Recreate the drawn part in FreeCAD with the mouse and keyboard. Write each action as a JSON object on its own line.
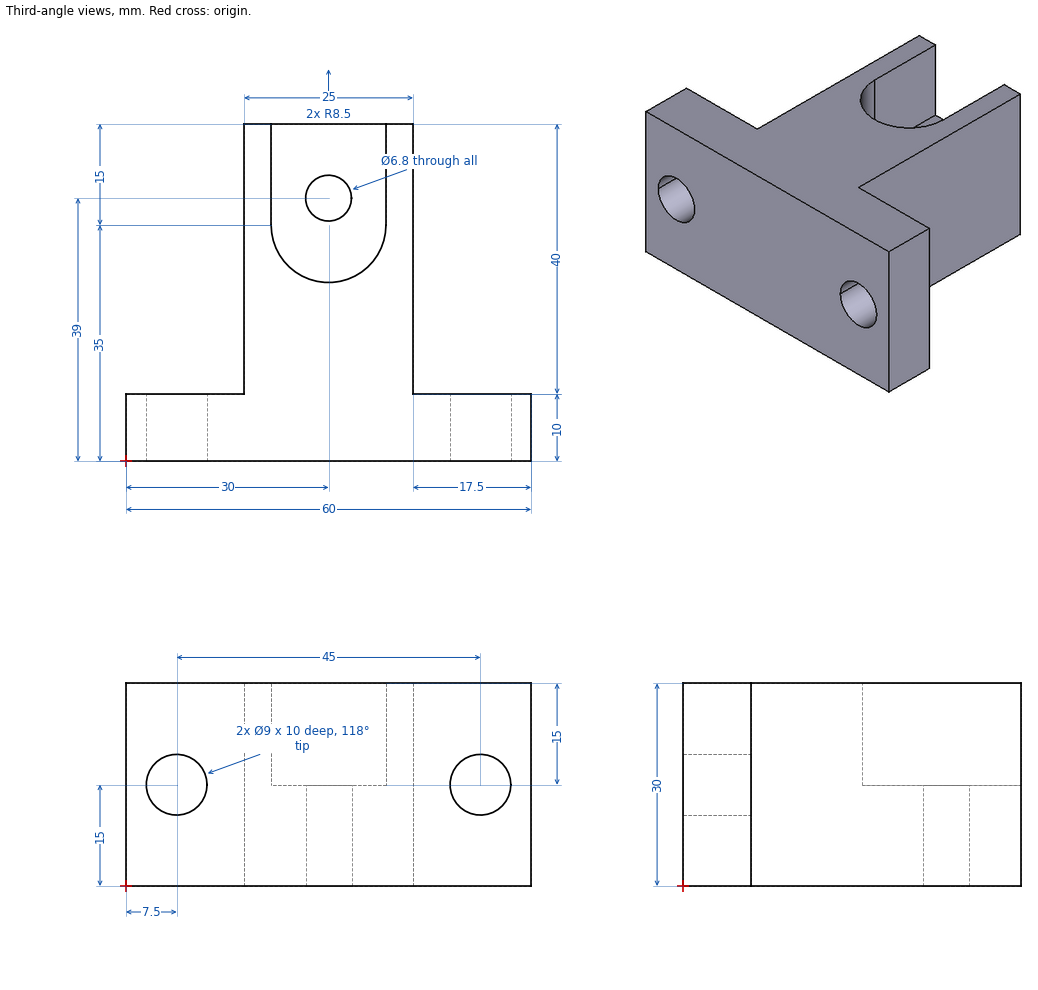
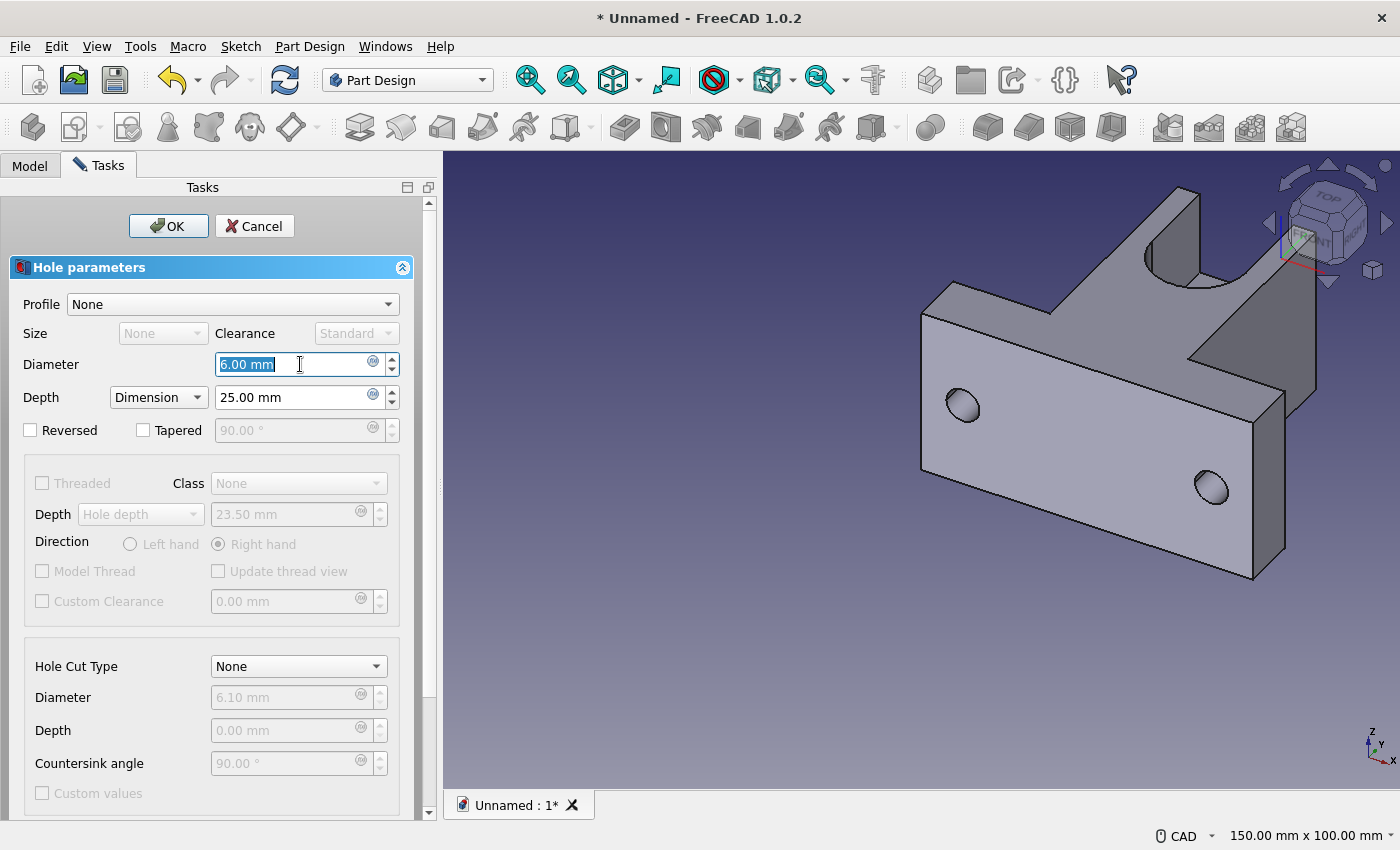
{"action": "type", "text": "9"}
{"action": "key", "text": "Tab"}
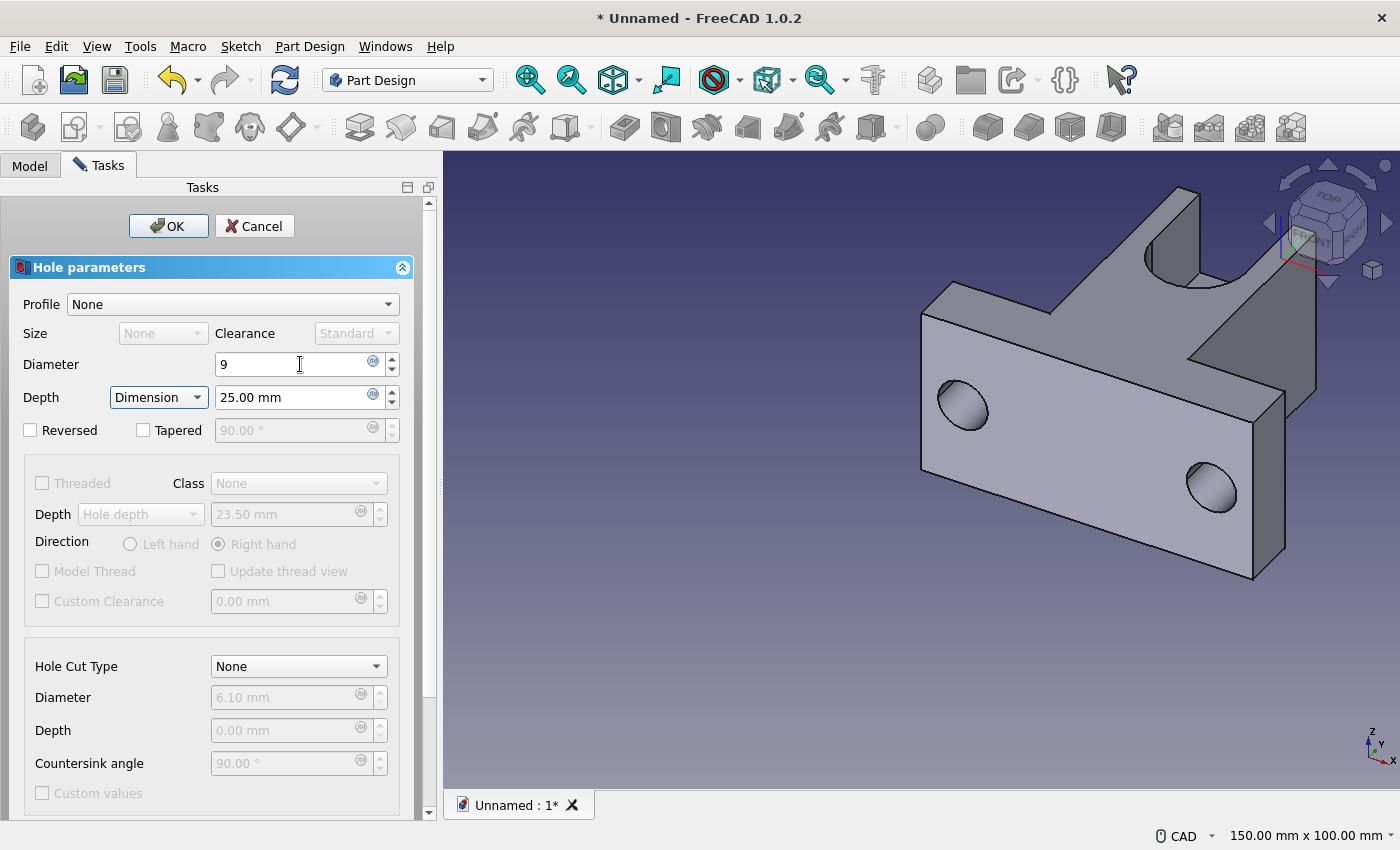
{"action": "triple_click", "coordinate": [300, 398]}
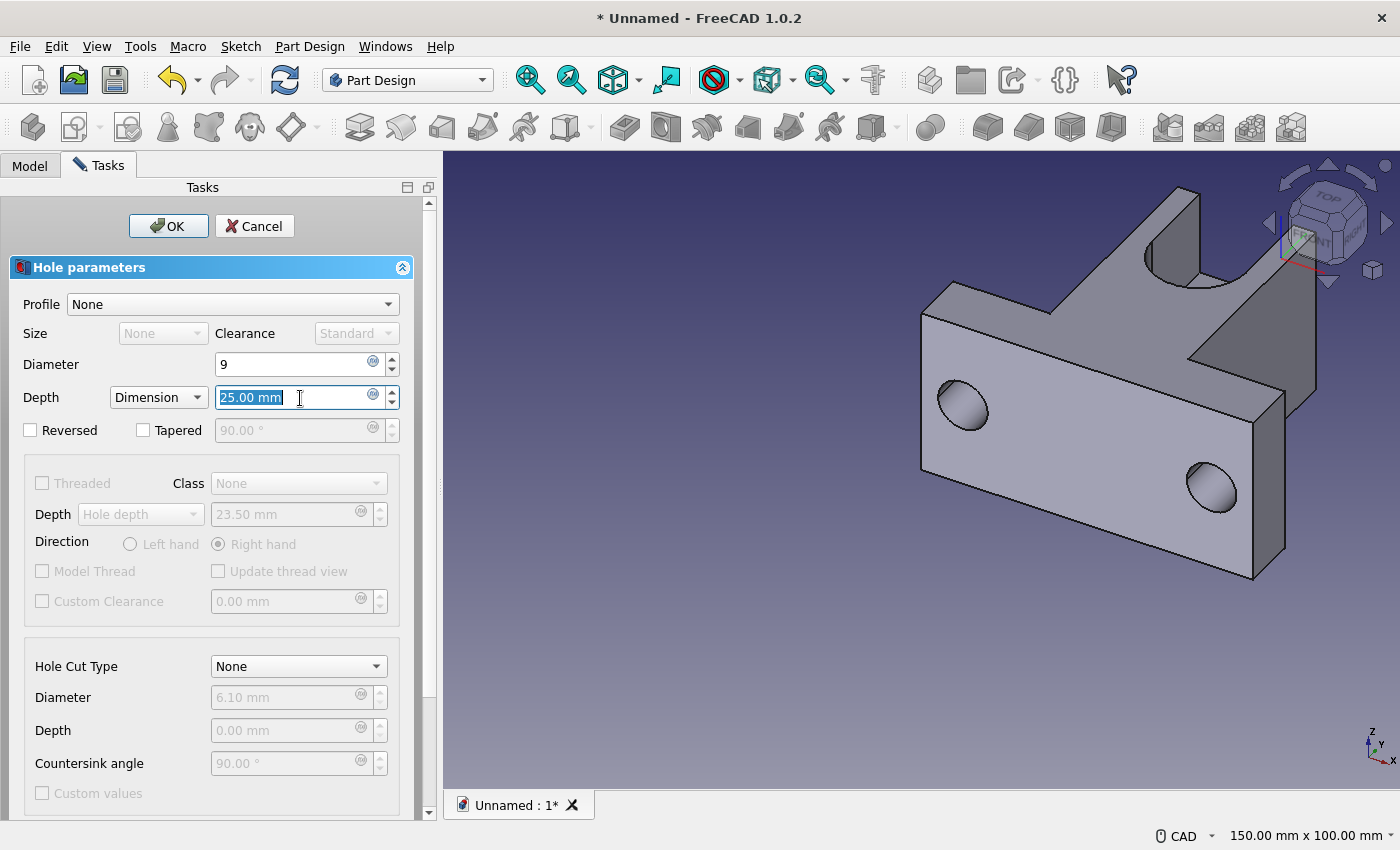
{"action": "type", "text": "10"}
{"action": "key", "text": "Tab"}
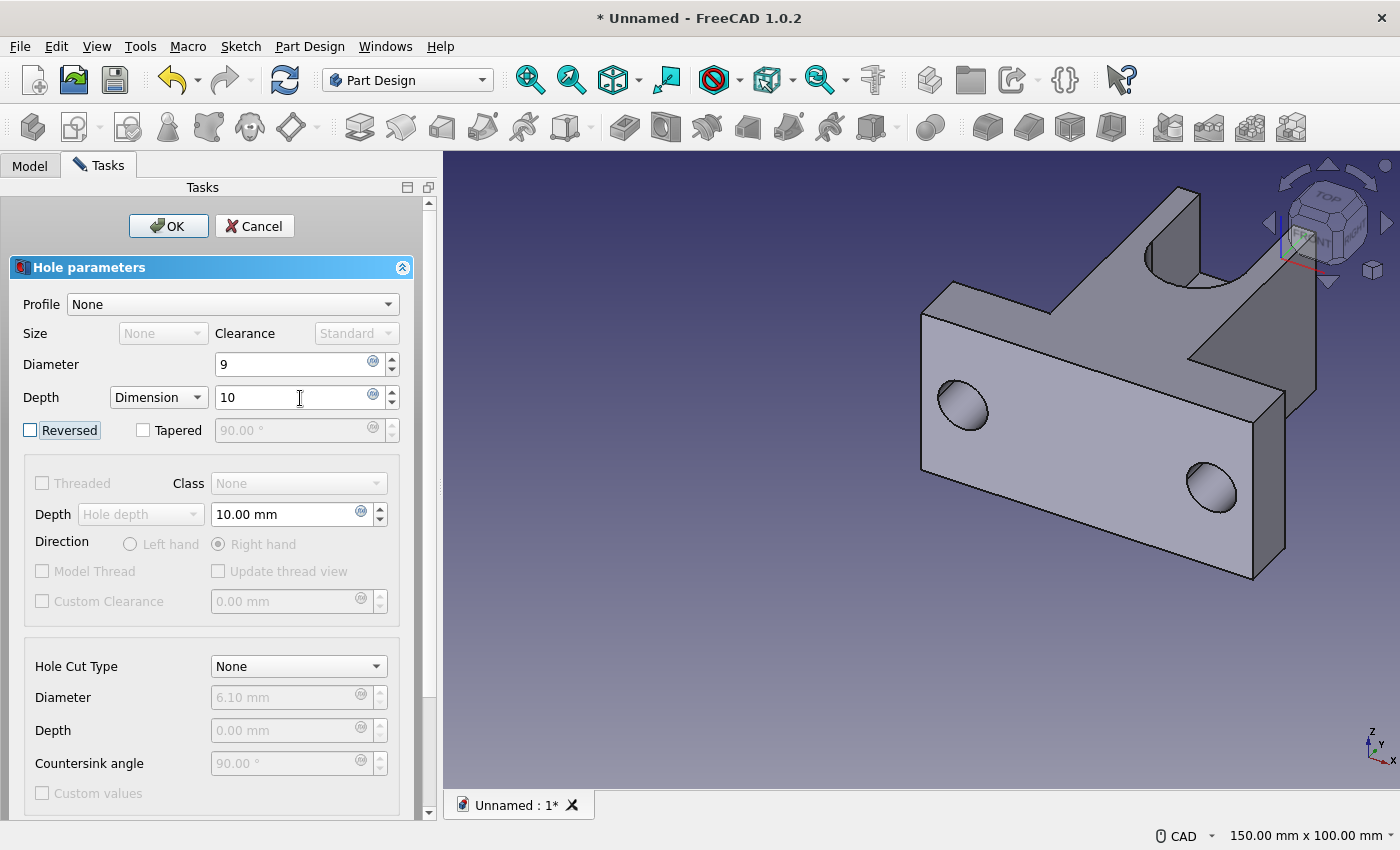
{"action": "left_click", "coordinate": [169, 226]}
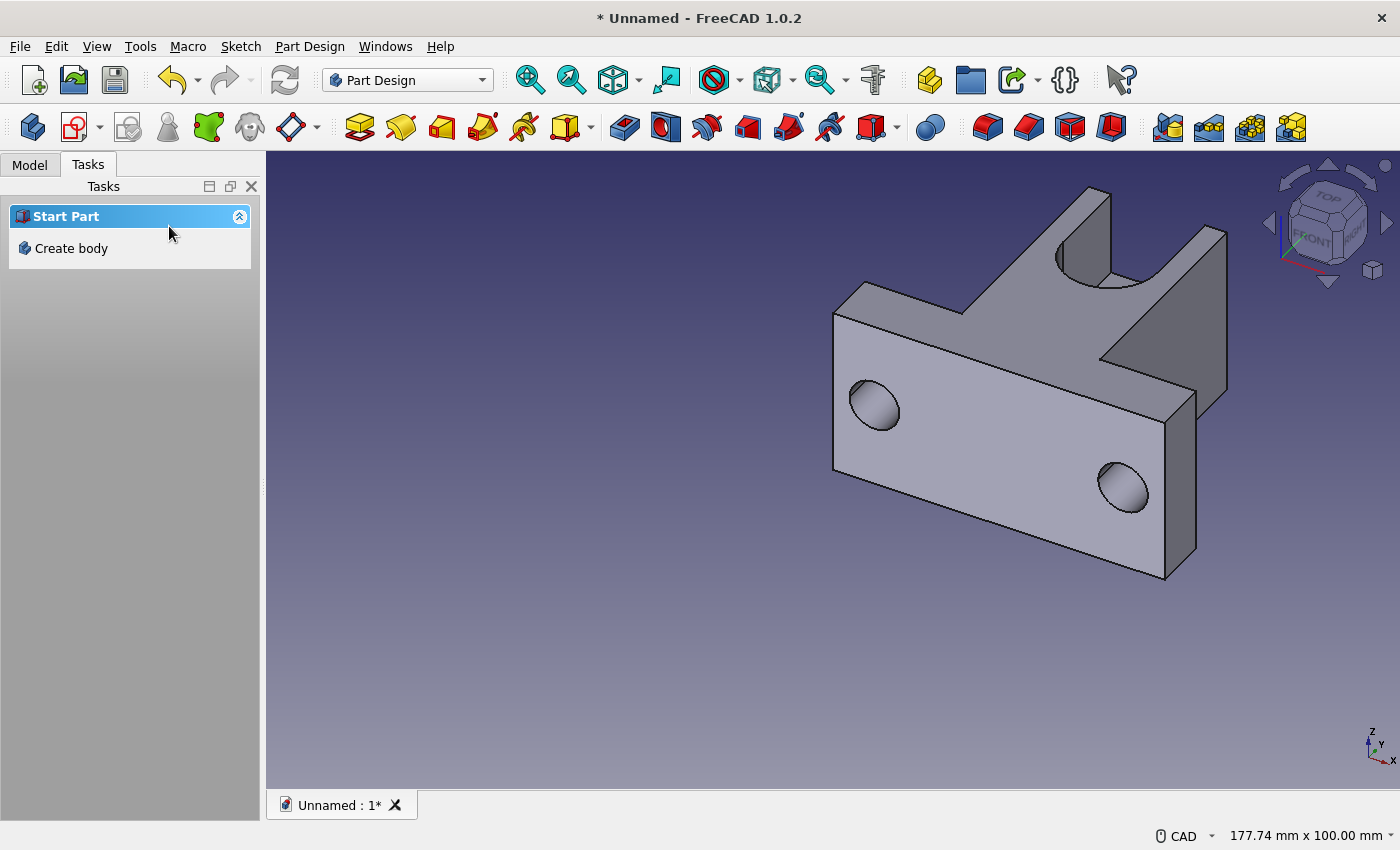
{"action": "left_click", "coordinate": [74, 128]}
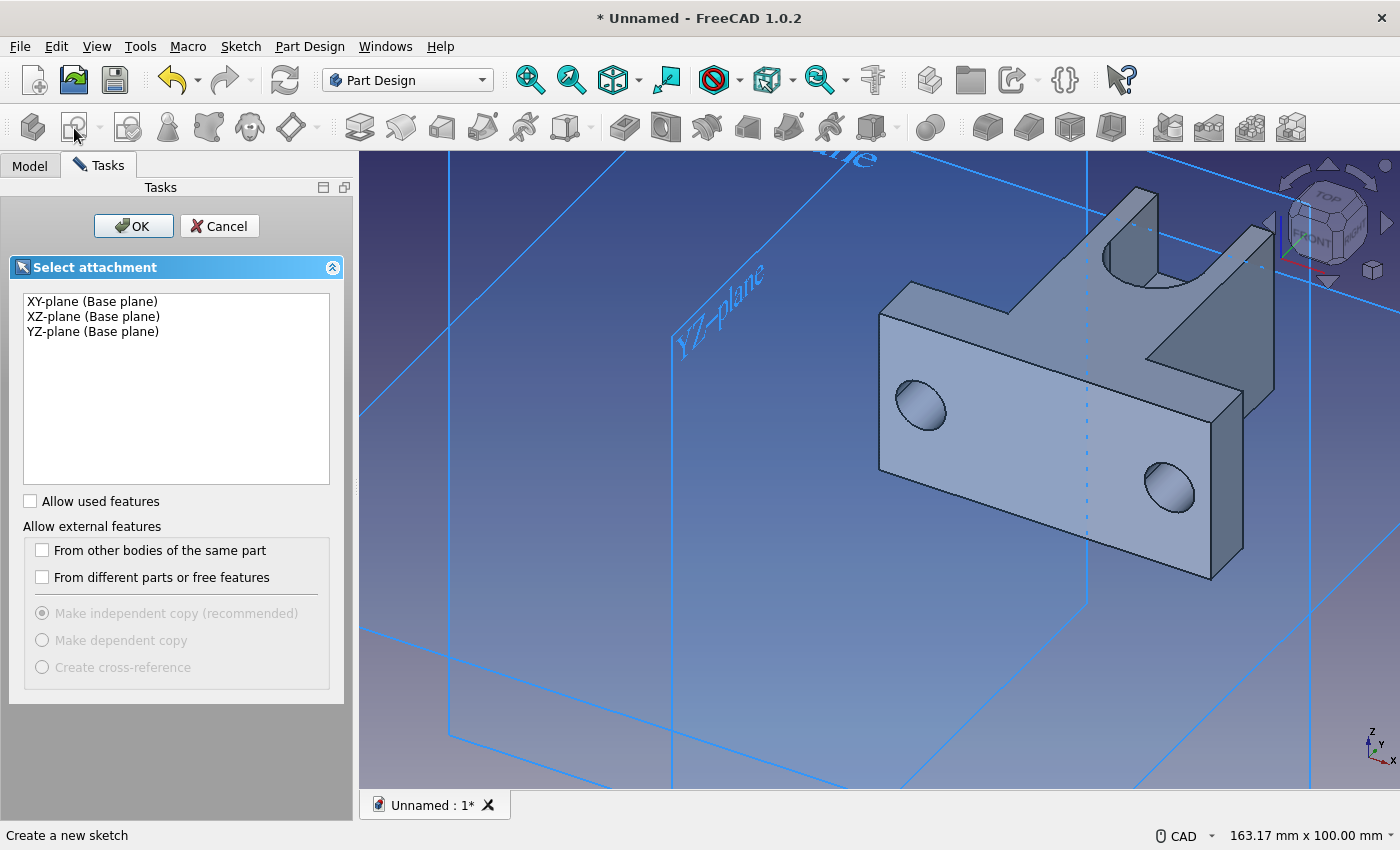
{"action": "left_click", "coordinate": [84, 302]}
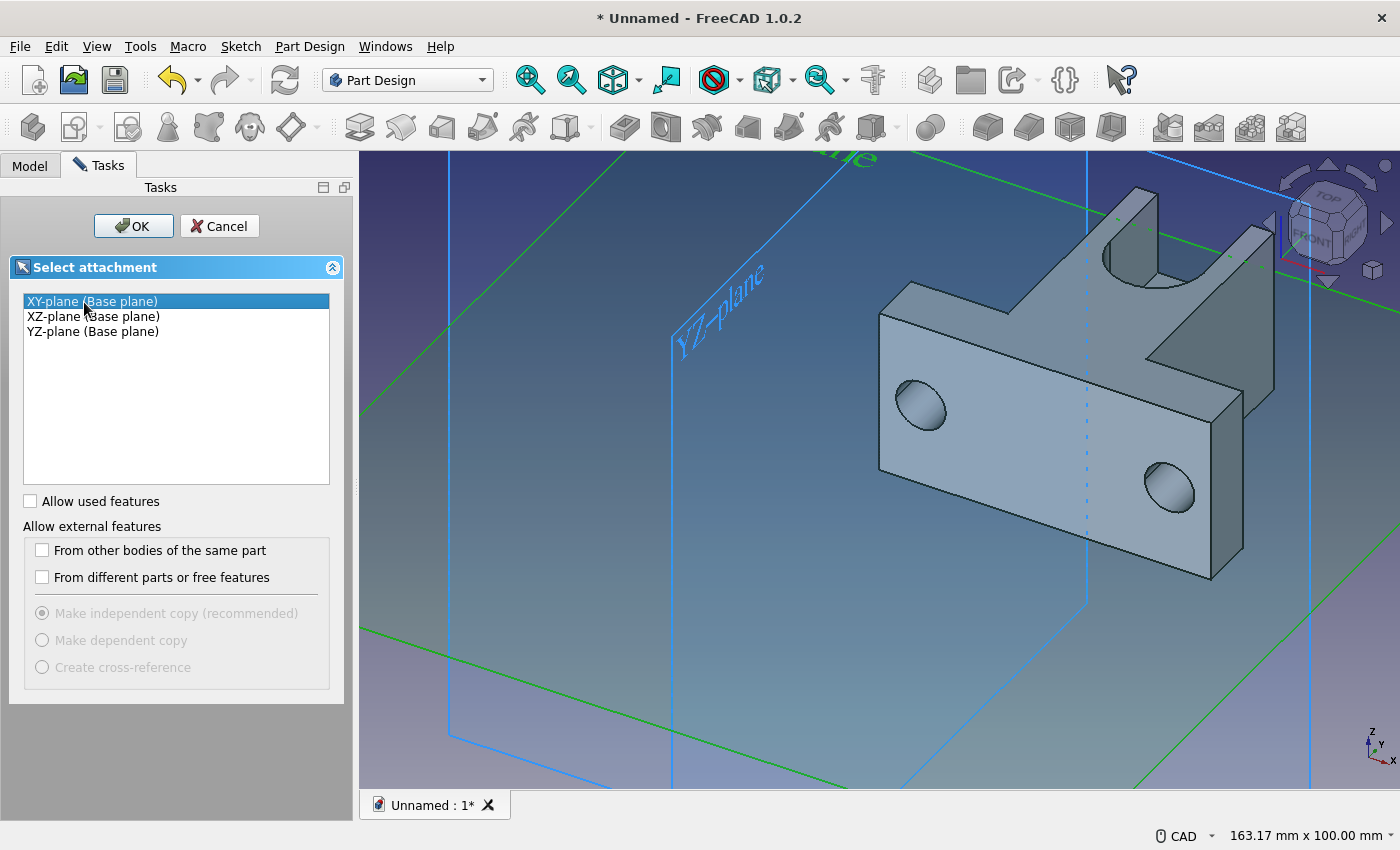
{"action": "left_click", "coordinate": [134, 226]}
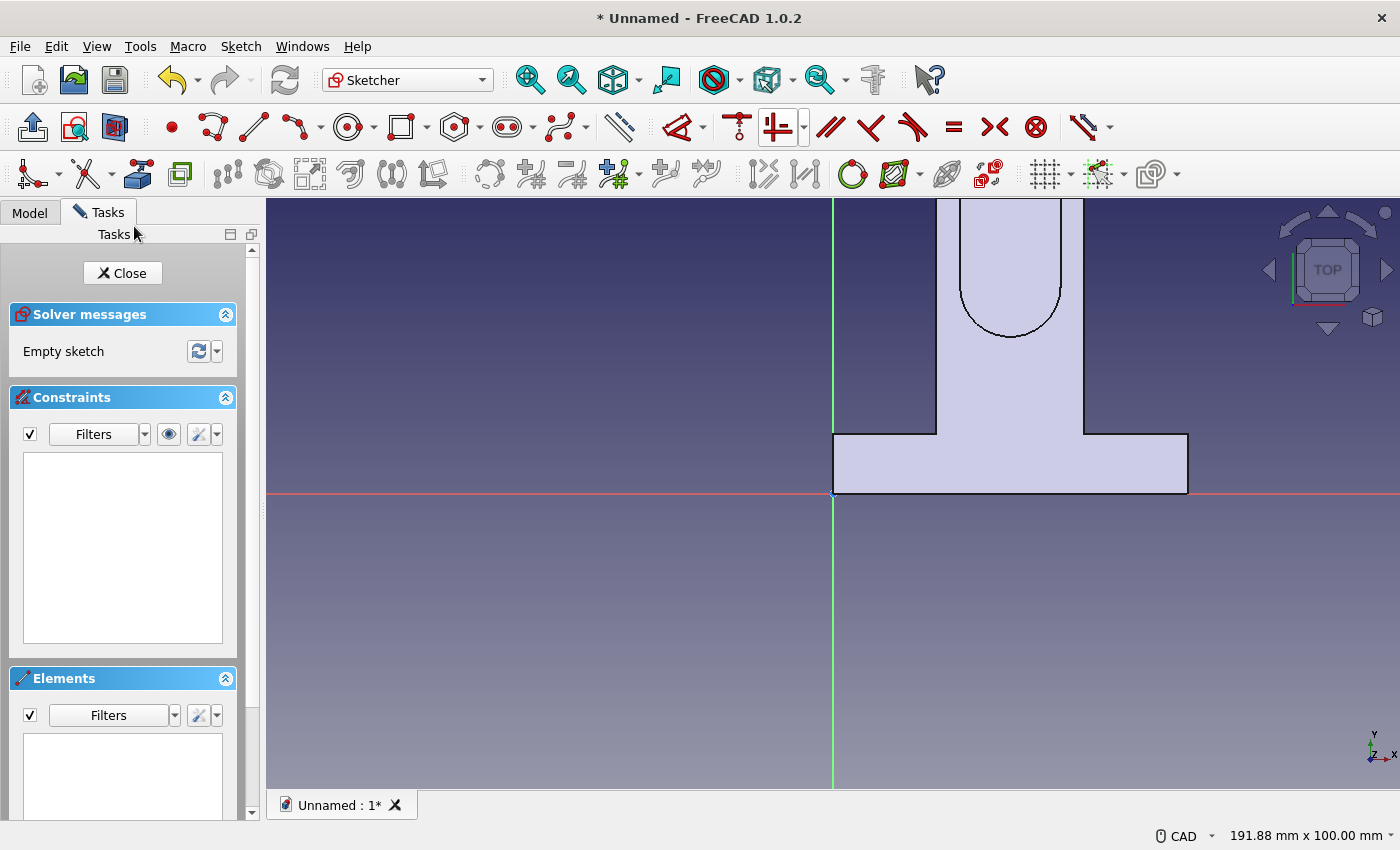
{"action": "key", "text": "q s"}